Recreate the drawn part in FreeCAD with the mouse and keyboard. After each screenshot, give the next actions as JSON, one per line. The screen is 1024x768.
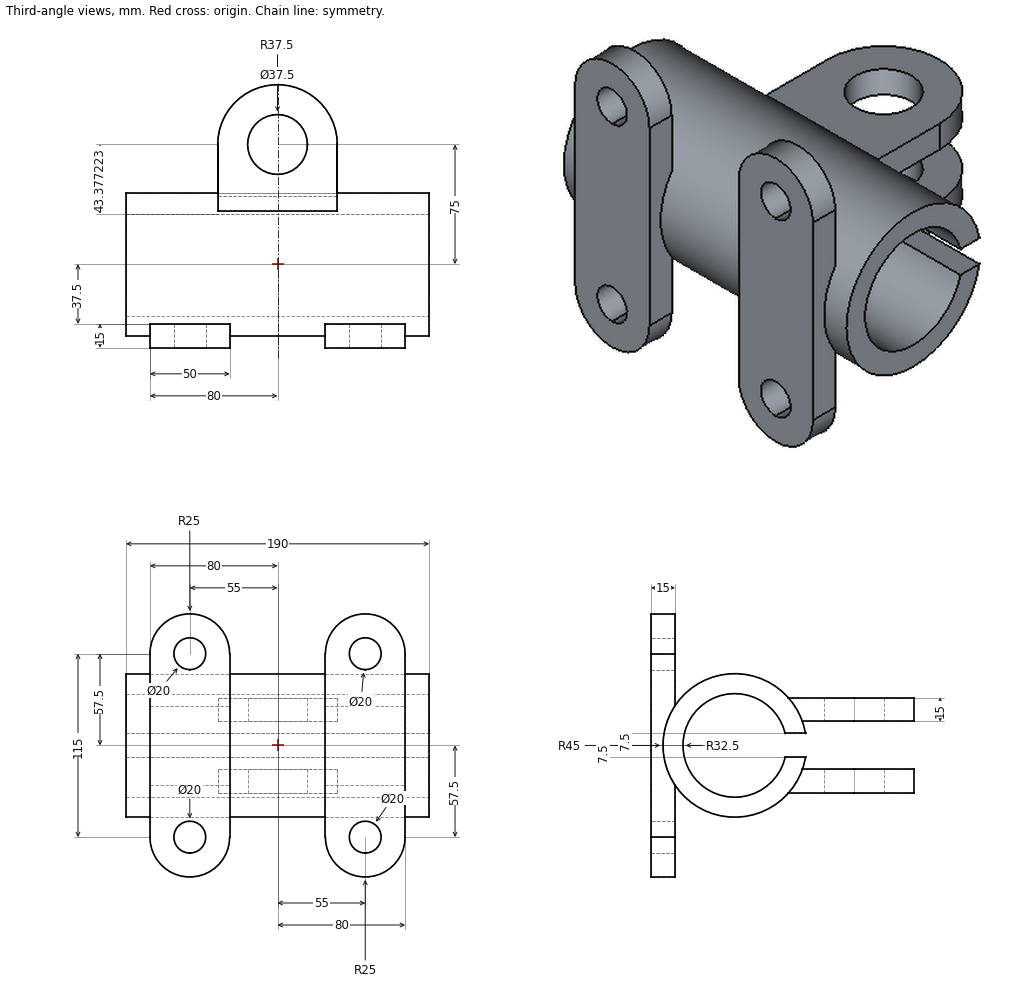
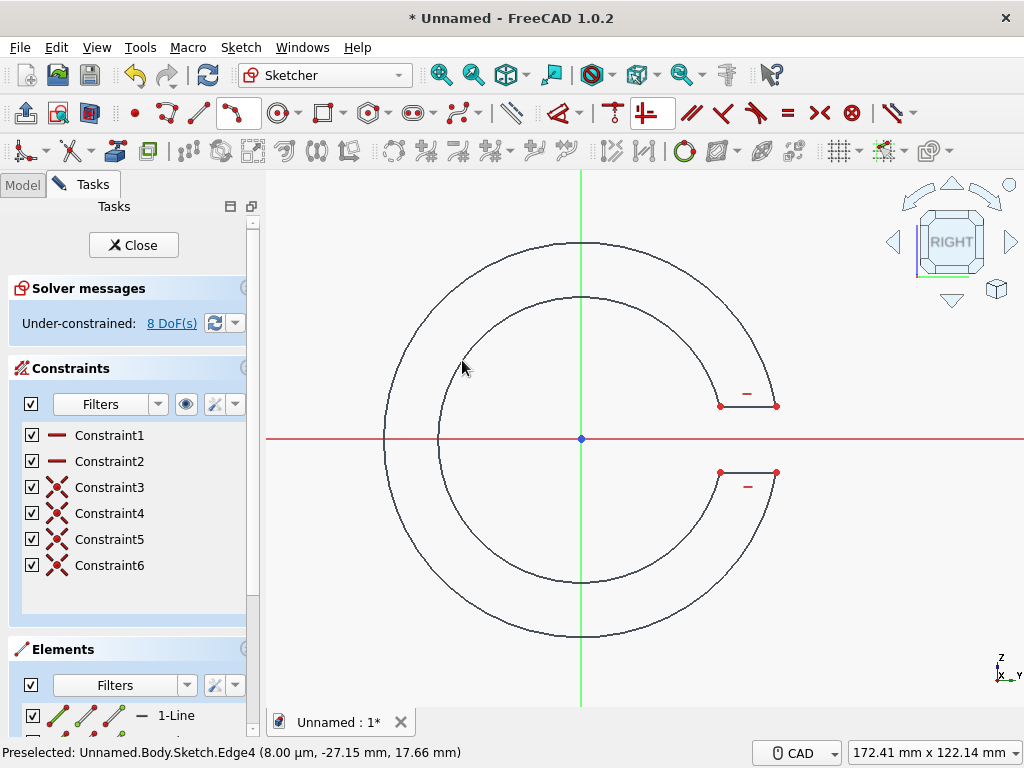
{"action": "left_click", "coordinate": [508, 257]}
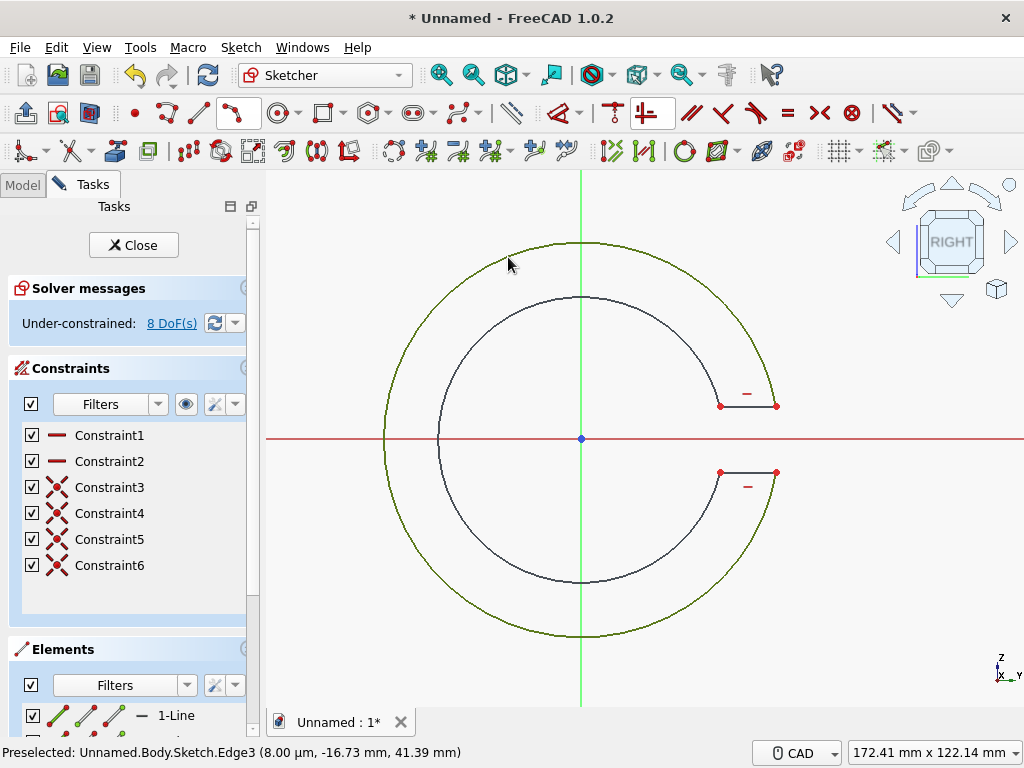
{"action": "left_click", "coordinate": [524, 309]}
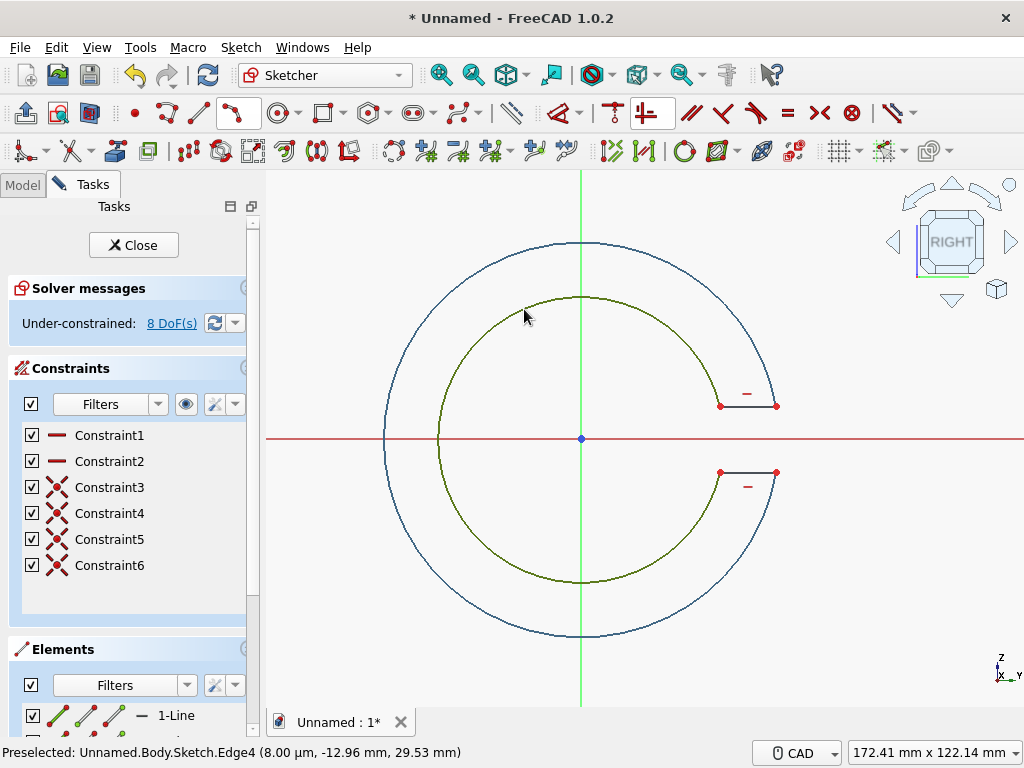
{"action": "left_click", "coordinate": [614, 114]}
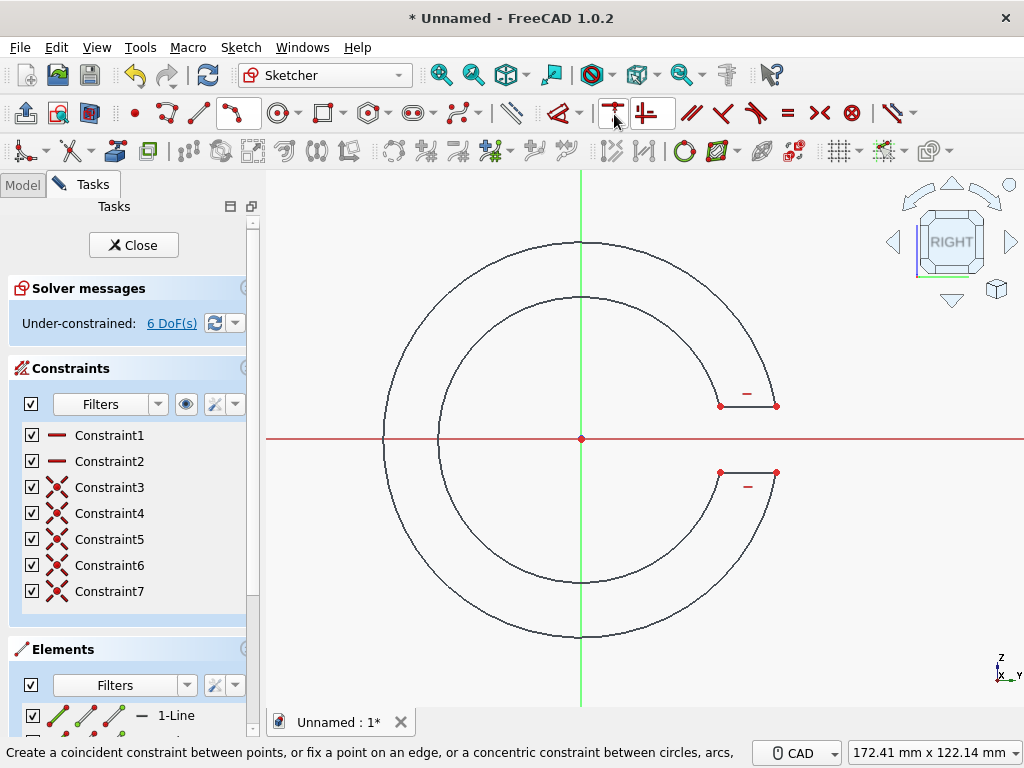
{"action": "left_click_drag", "start_coordinate": [571, 429], "coordinate": [591, 450]}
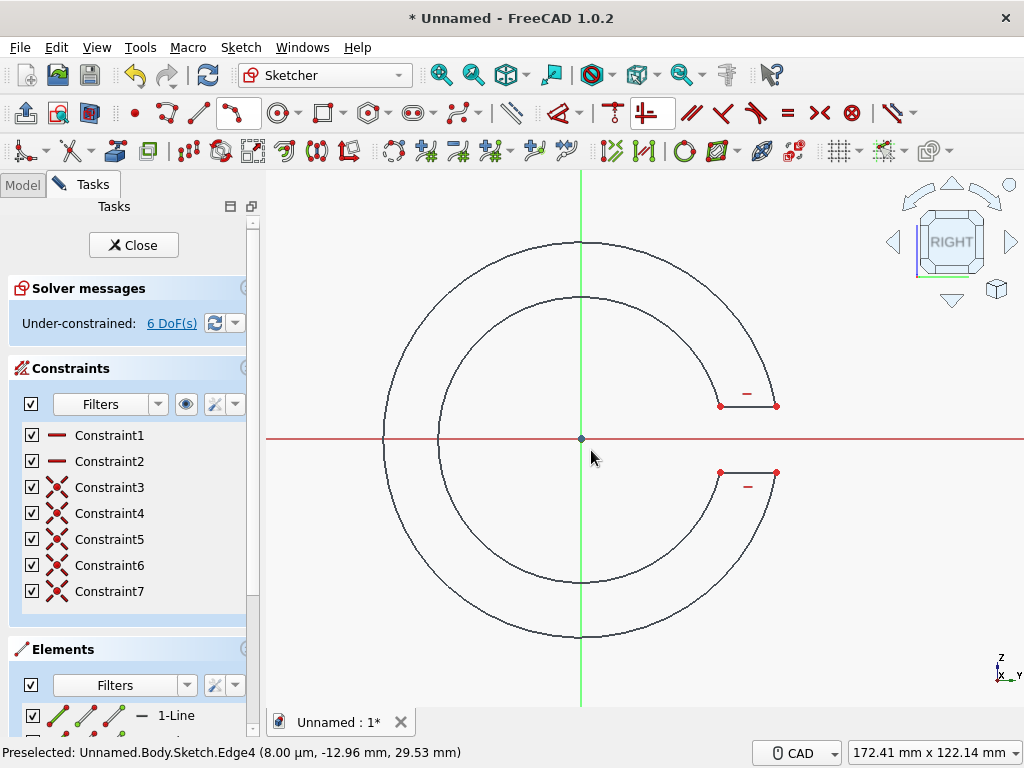
{"action": "left_click", "coordinate": [614, 114]}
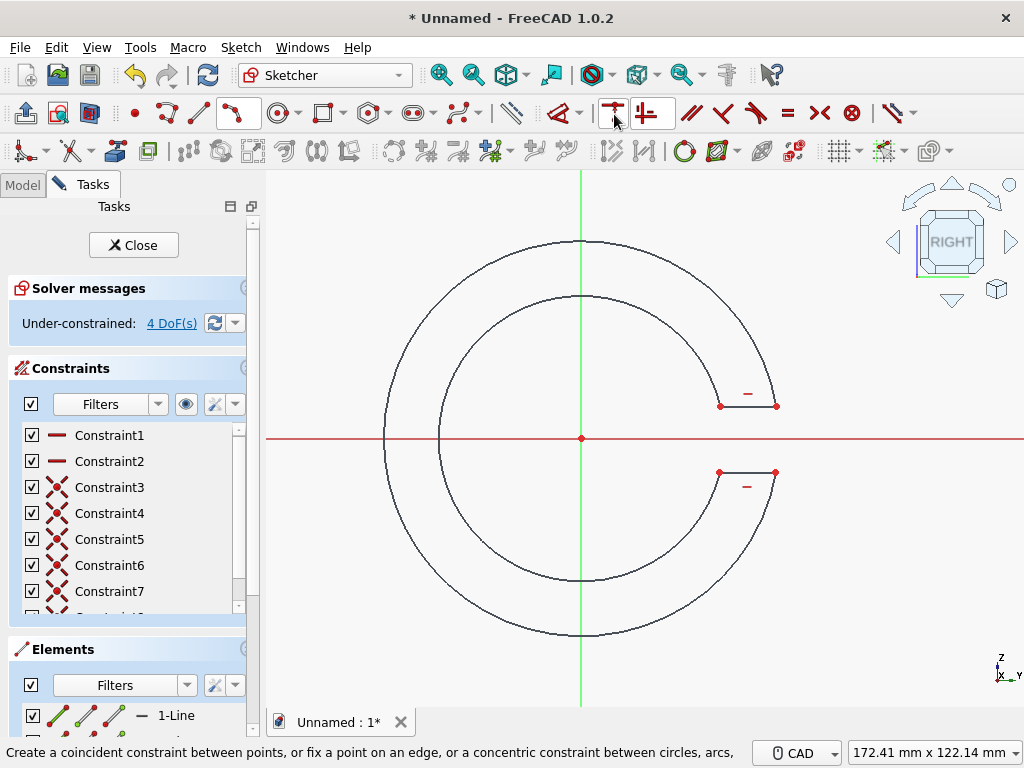
{"action": "left_click", "coordinate": [509, 255]}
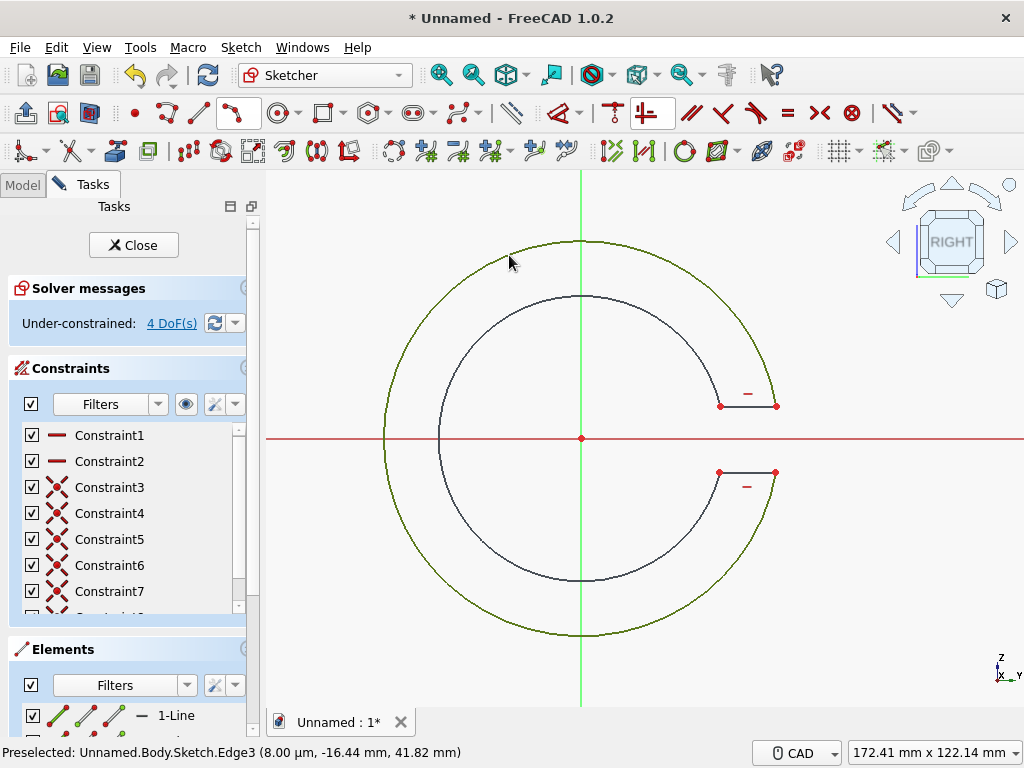
{"action": "left_click", "coordinate": [582, 114]}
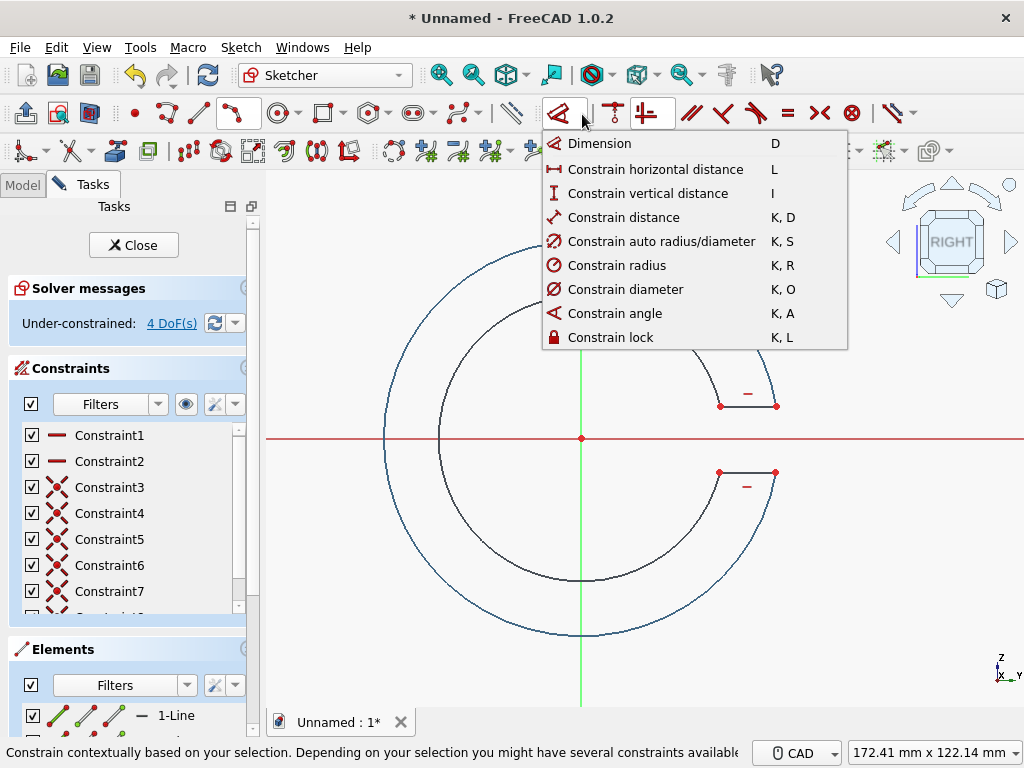
{"action": "left_click", "coordinate": [695, 265]}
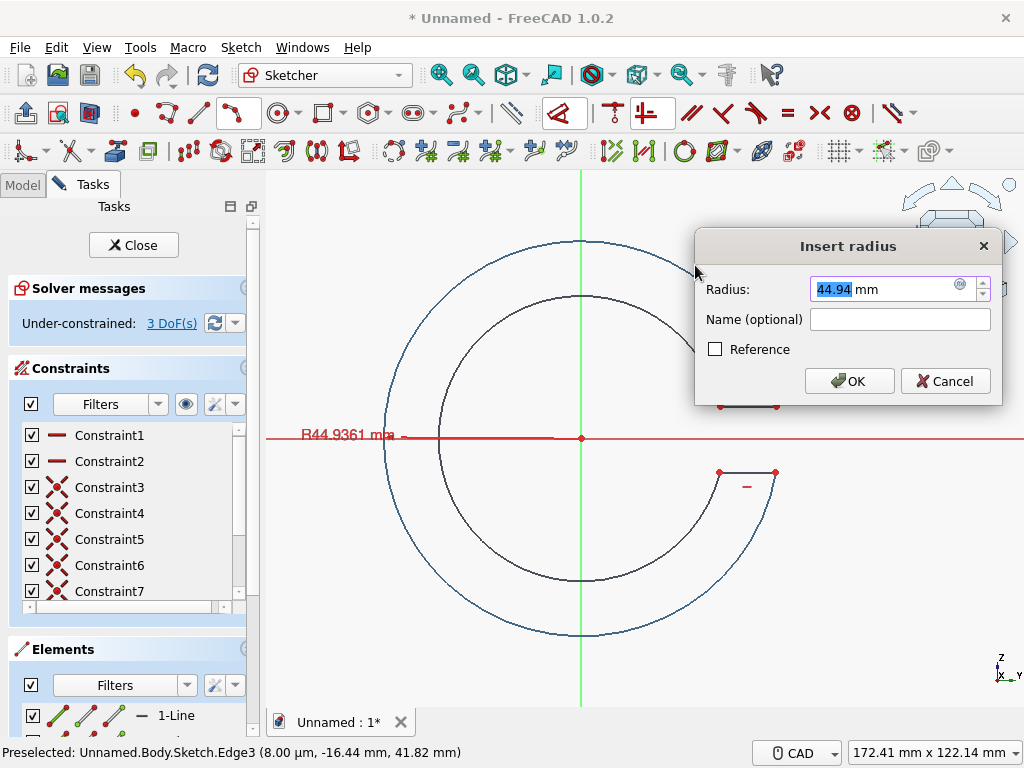
{"action": "type", "text": "45"}
{"action": "key", "text": "Return"}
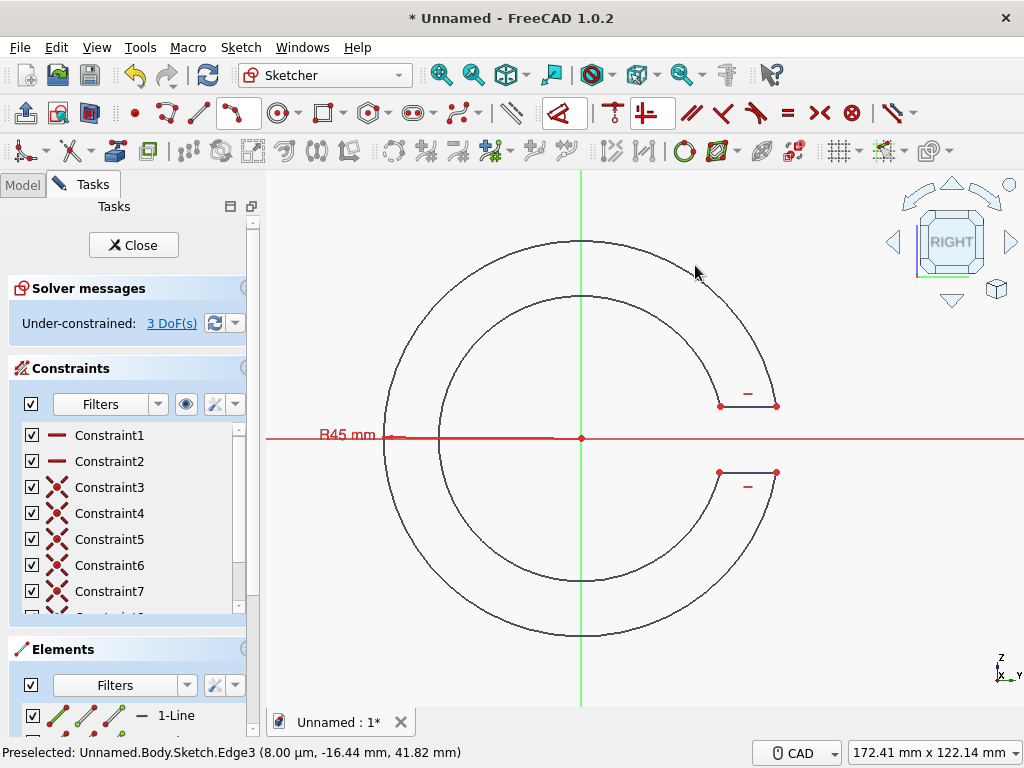
{"action": "left_click", "coordinate": [526, 307]}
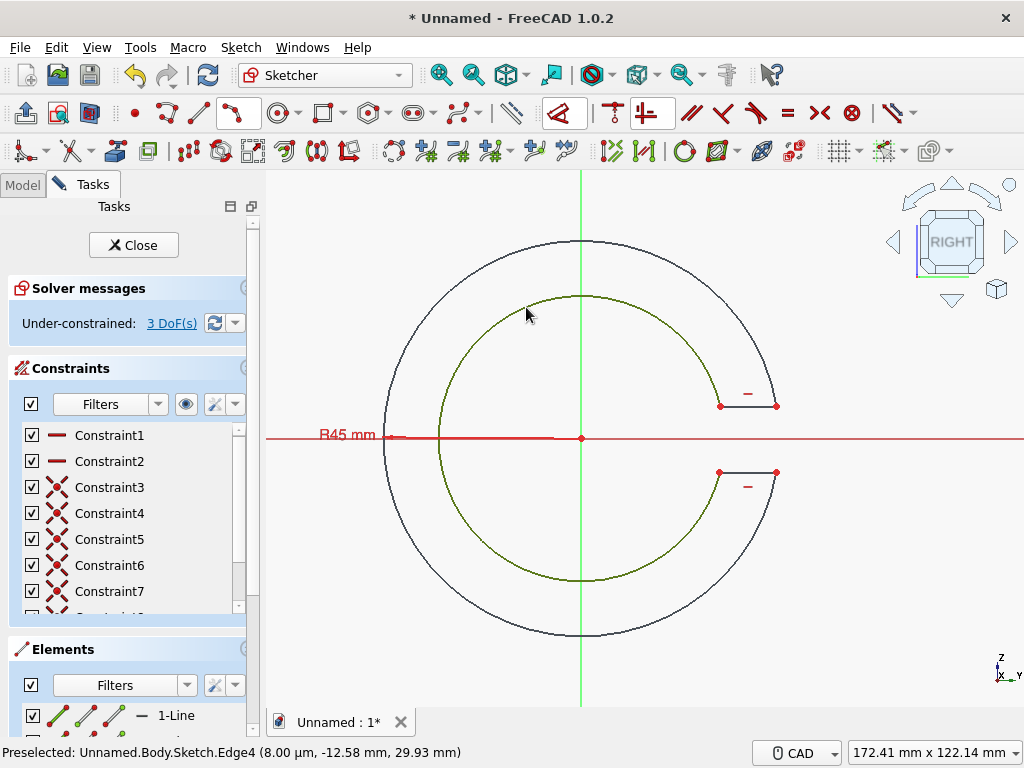
{"action": "left_click", "coordinate": [582, 114]}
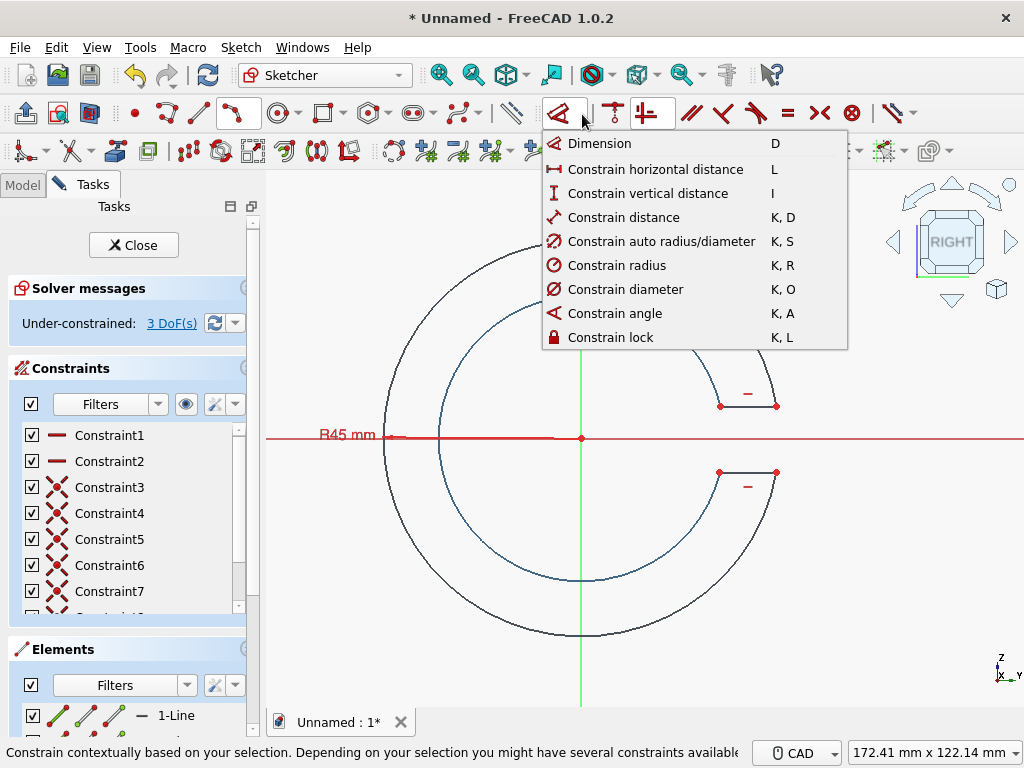
{"action": "left_click", "coordinate": [695, 265]}